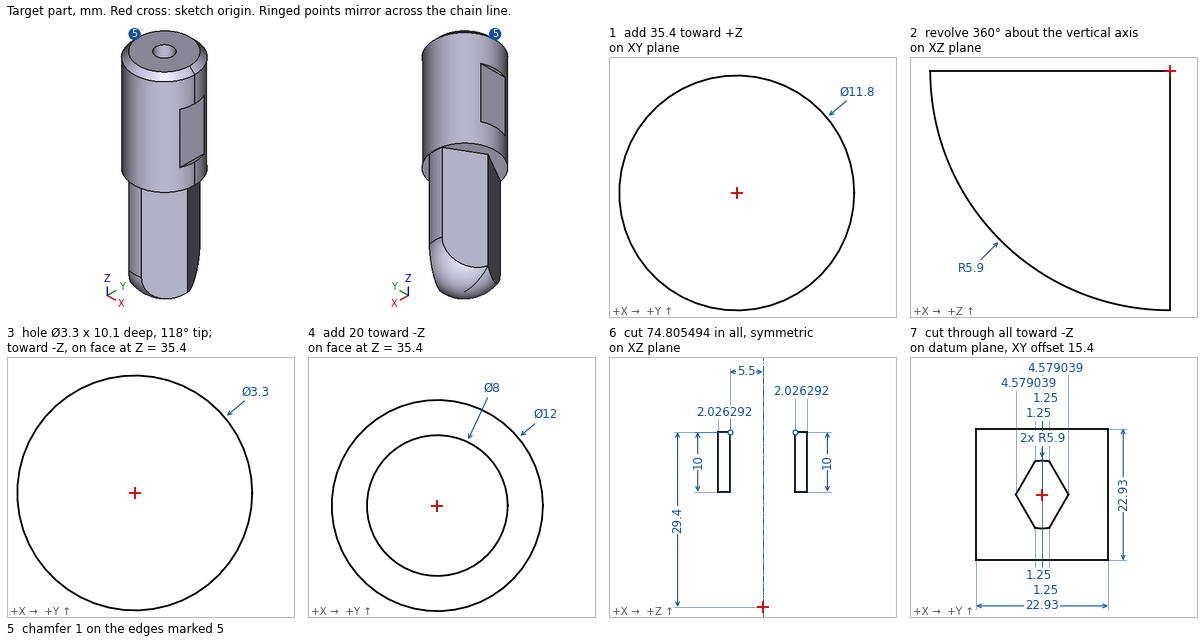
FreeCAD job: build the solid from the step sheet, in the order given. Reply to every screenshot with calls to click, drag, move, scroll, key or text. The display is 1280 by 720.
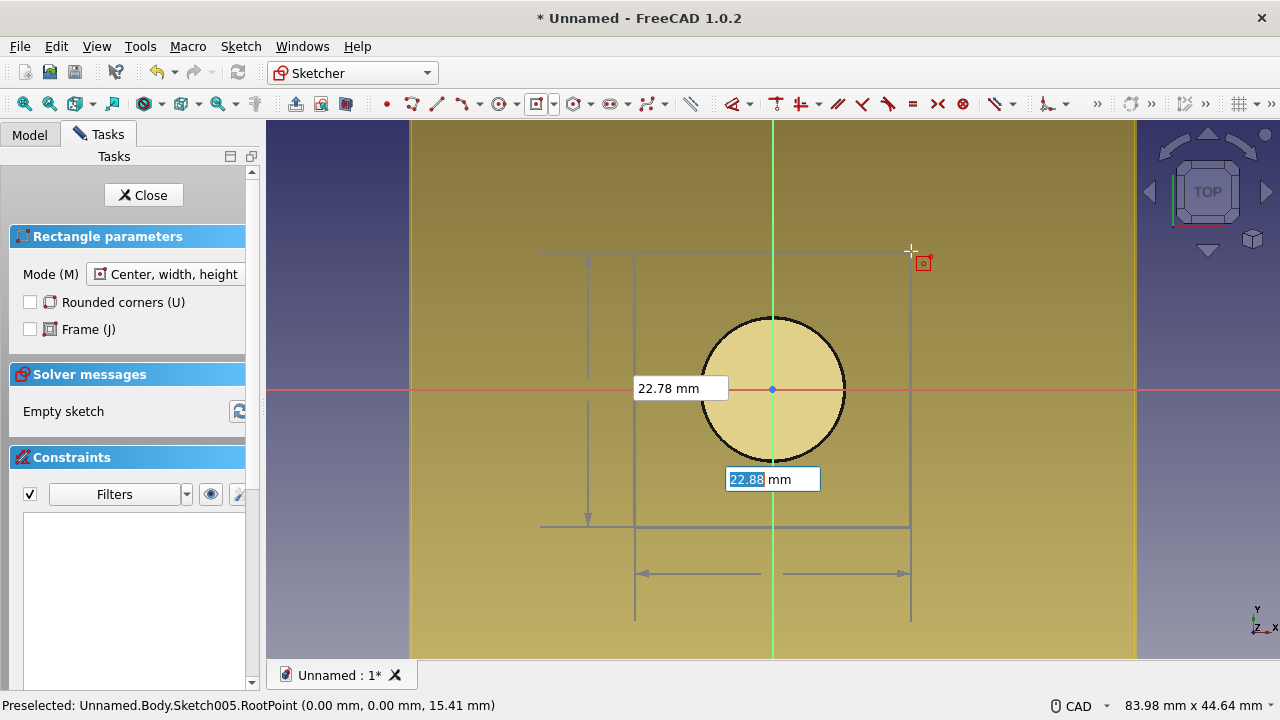
text(22.93)
key(Tab)
text(22.93)
key(Return)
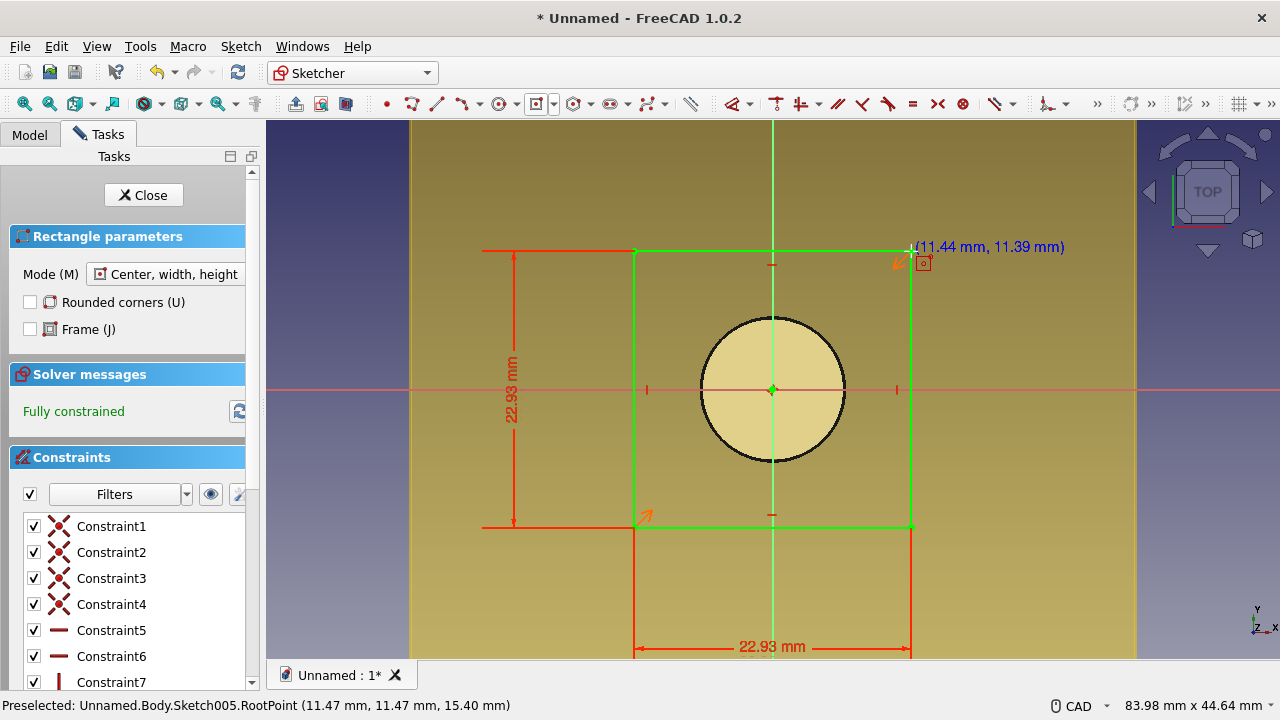
key(g)
key(m)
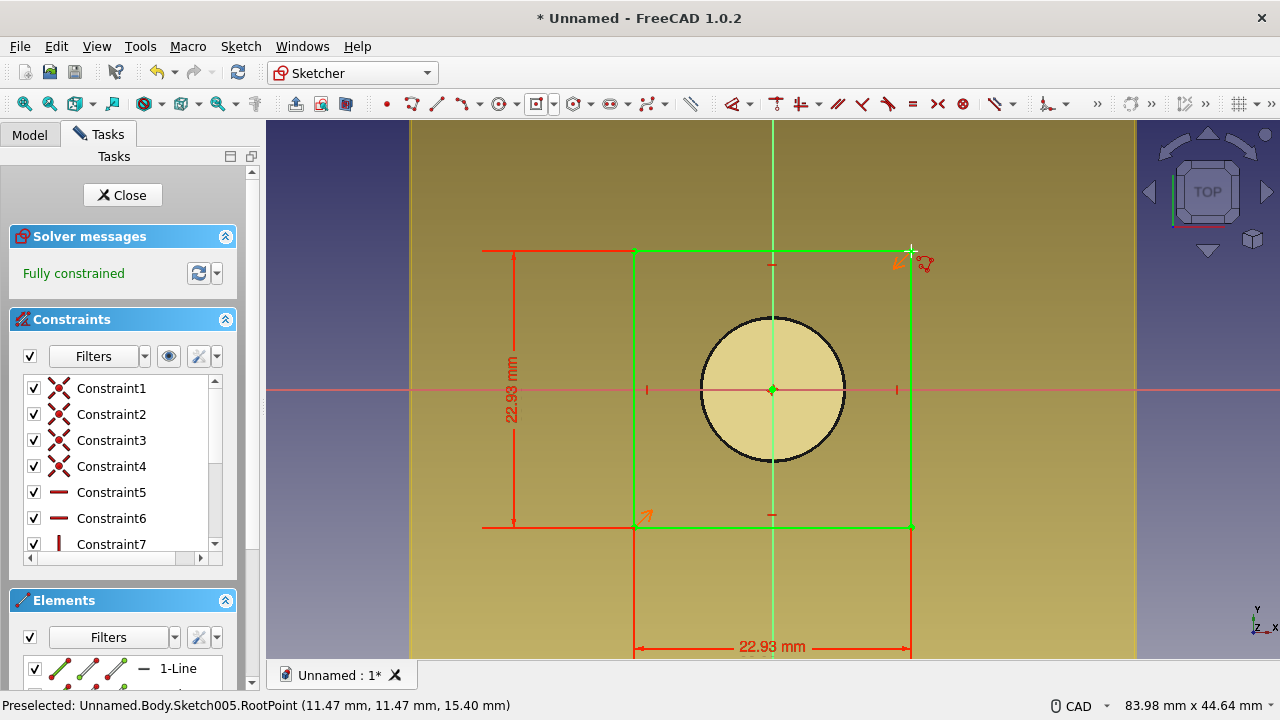
click(758, 320)
click(718, 390)
click(758, 459)
right_click(758, 459)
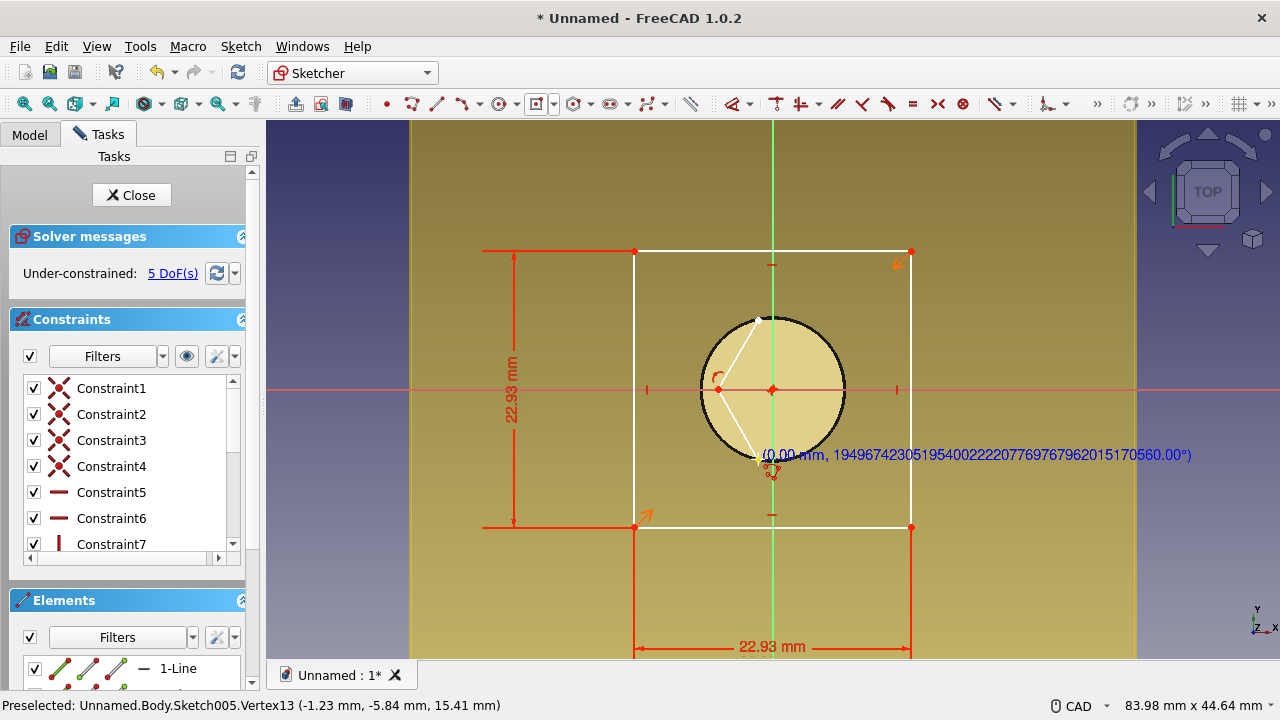
click(788, 459)
click(828, 390)
click(788, 320)
right_click(788, 320)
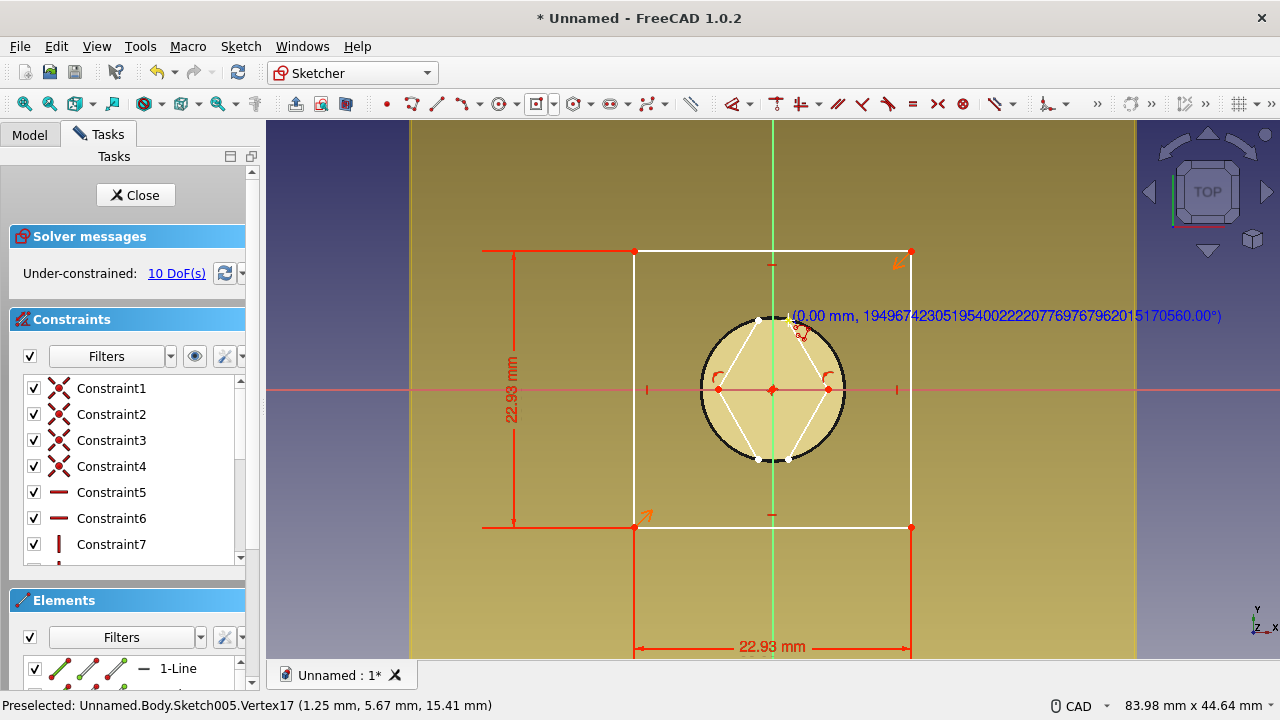
key(g)
key(3)
key(a)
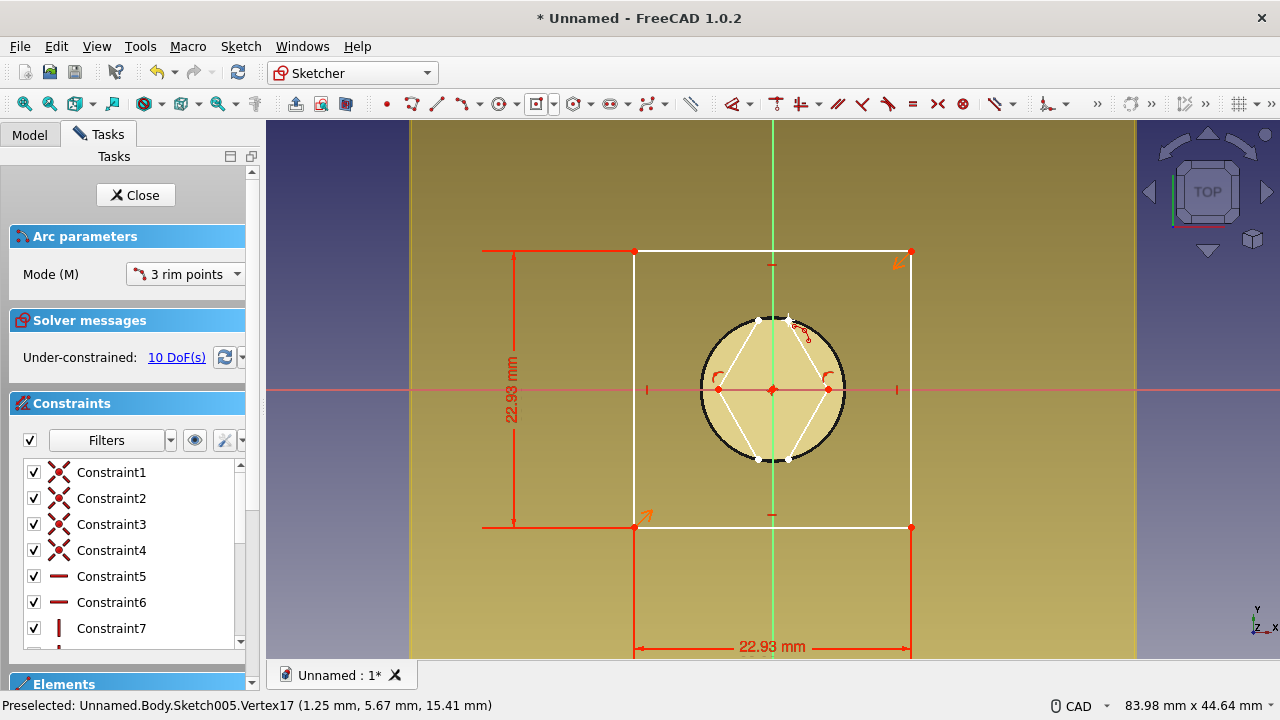
click(758, 460)
click(788, 460)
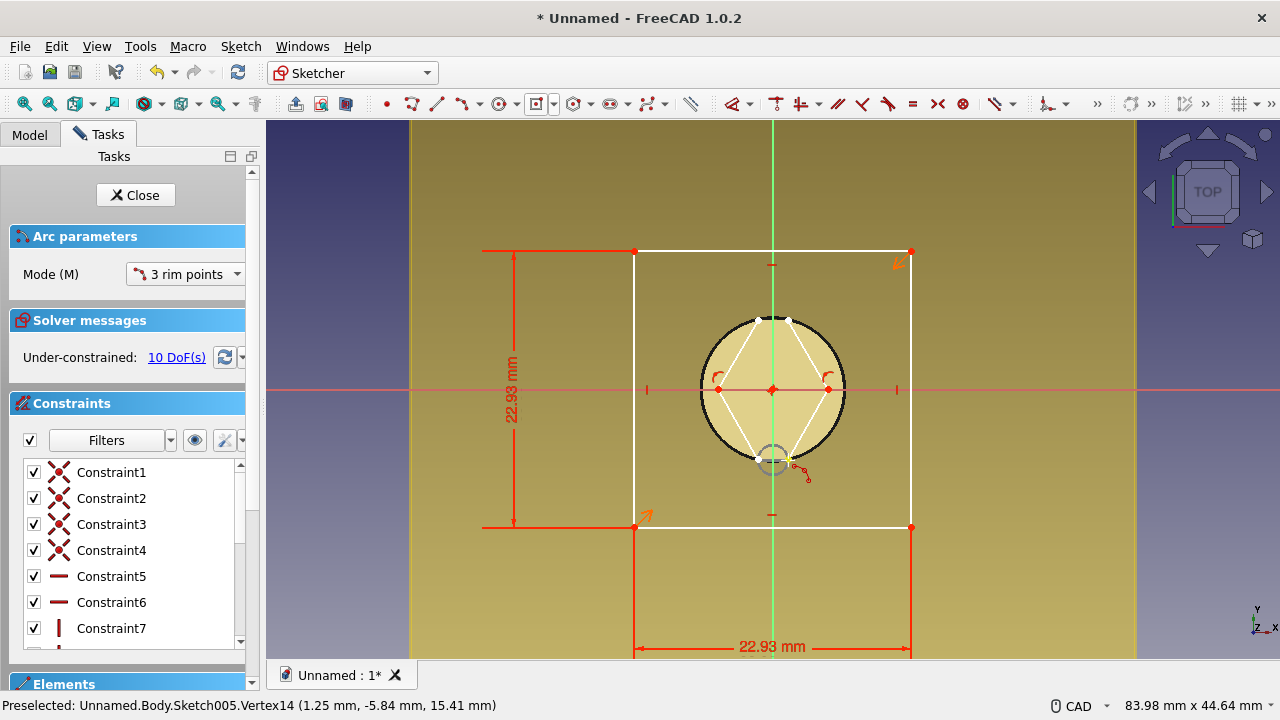
scroll(770, 461, up, 12)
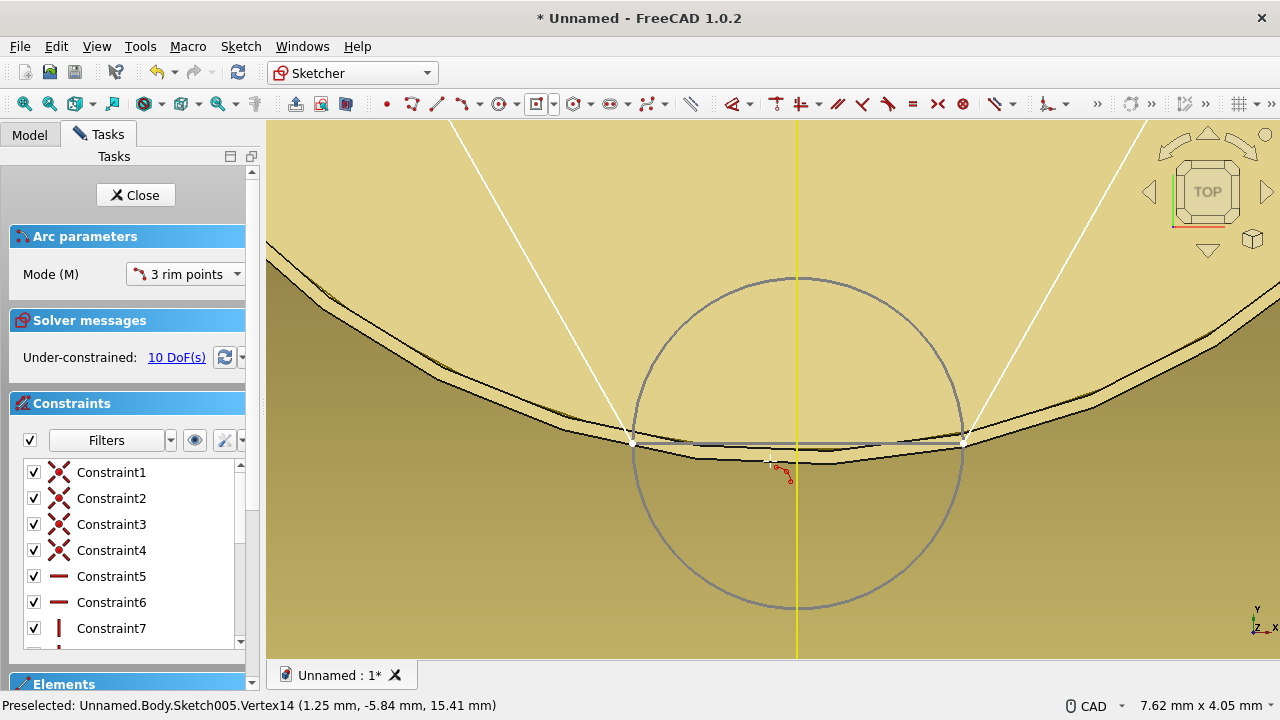
click(763, 451)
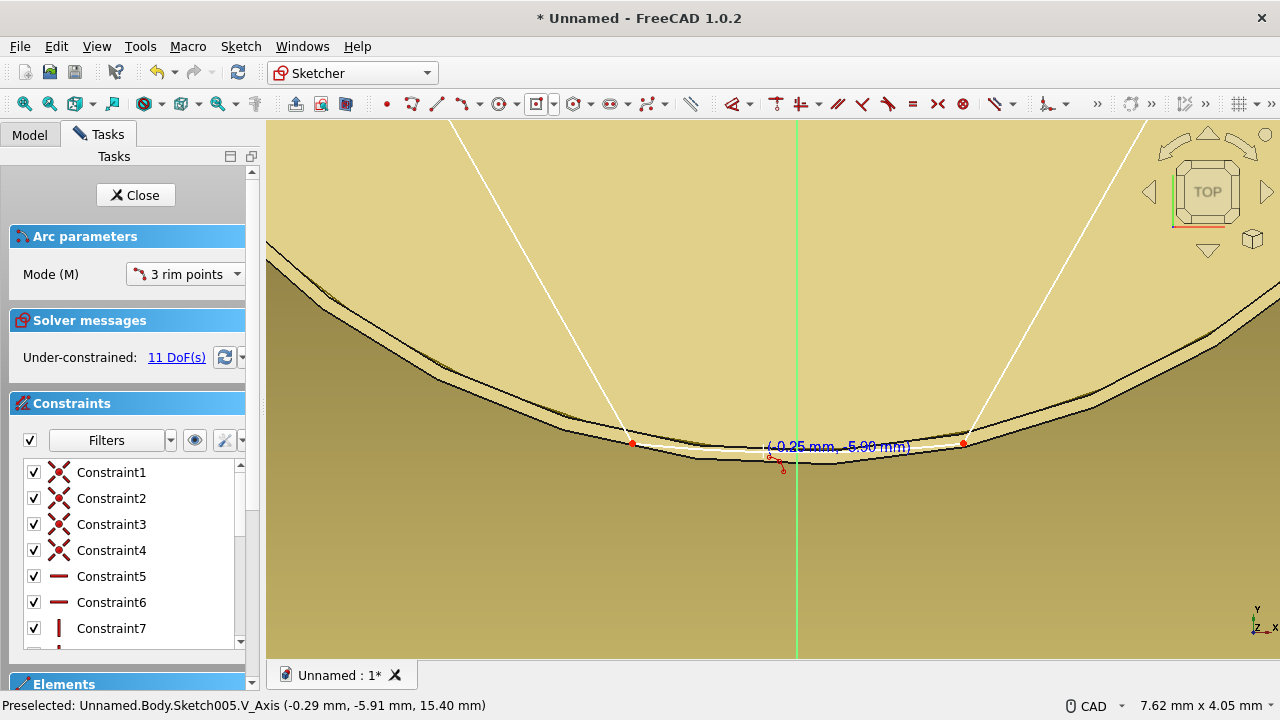
scroll(693, 480, down, 11)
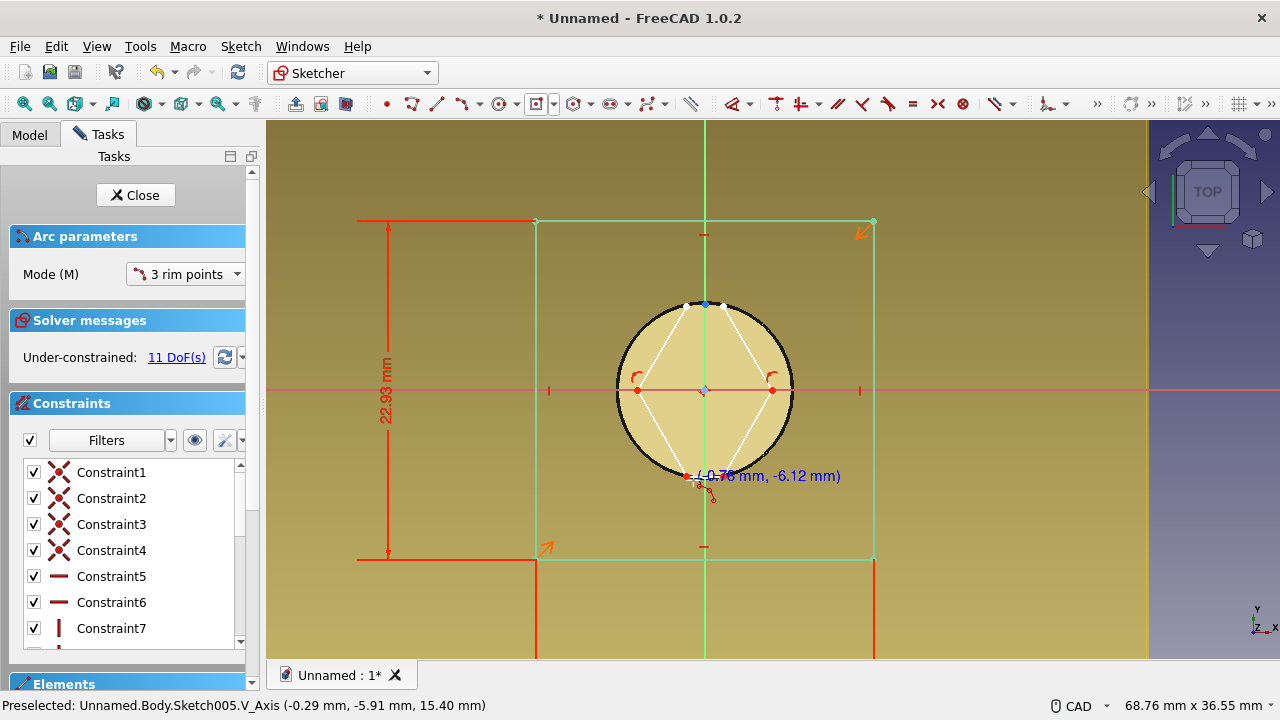
click(723, 307)
click(687, 307)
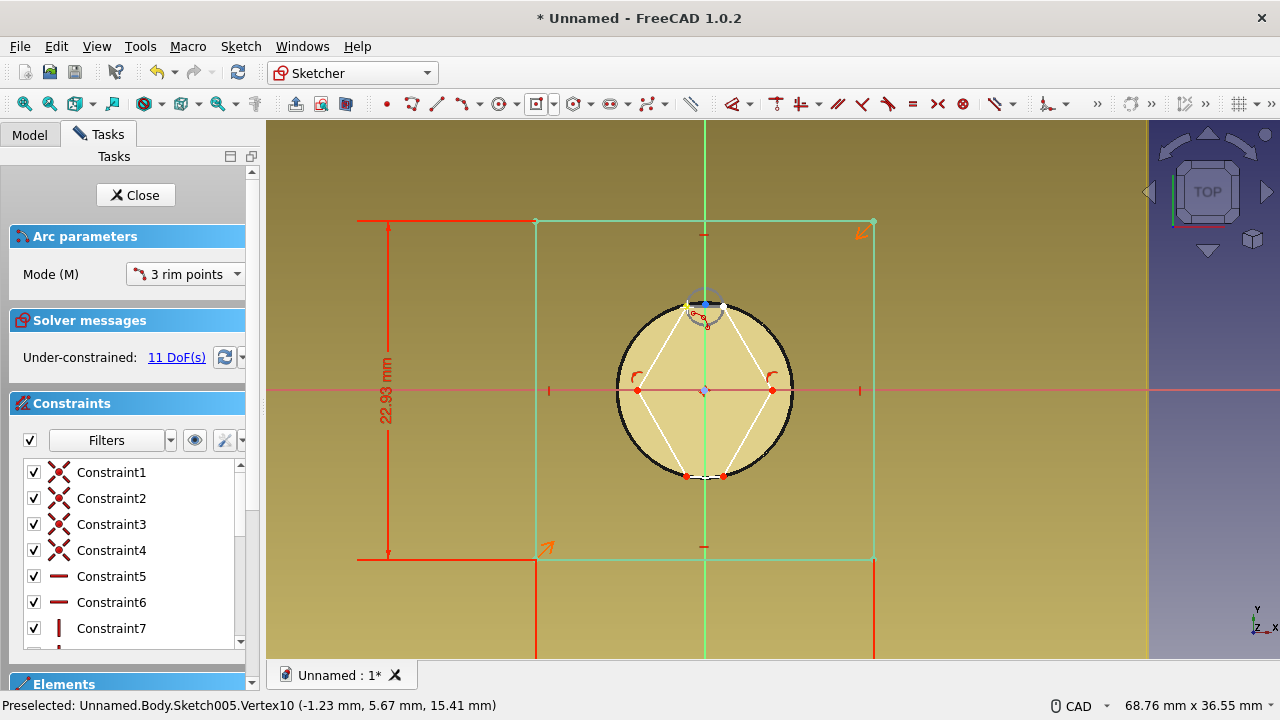
scroll(709, 304, up, 11)